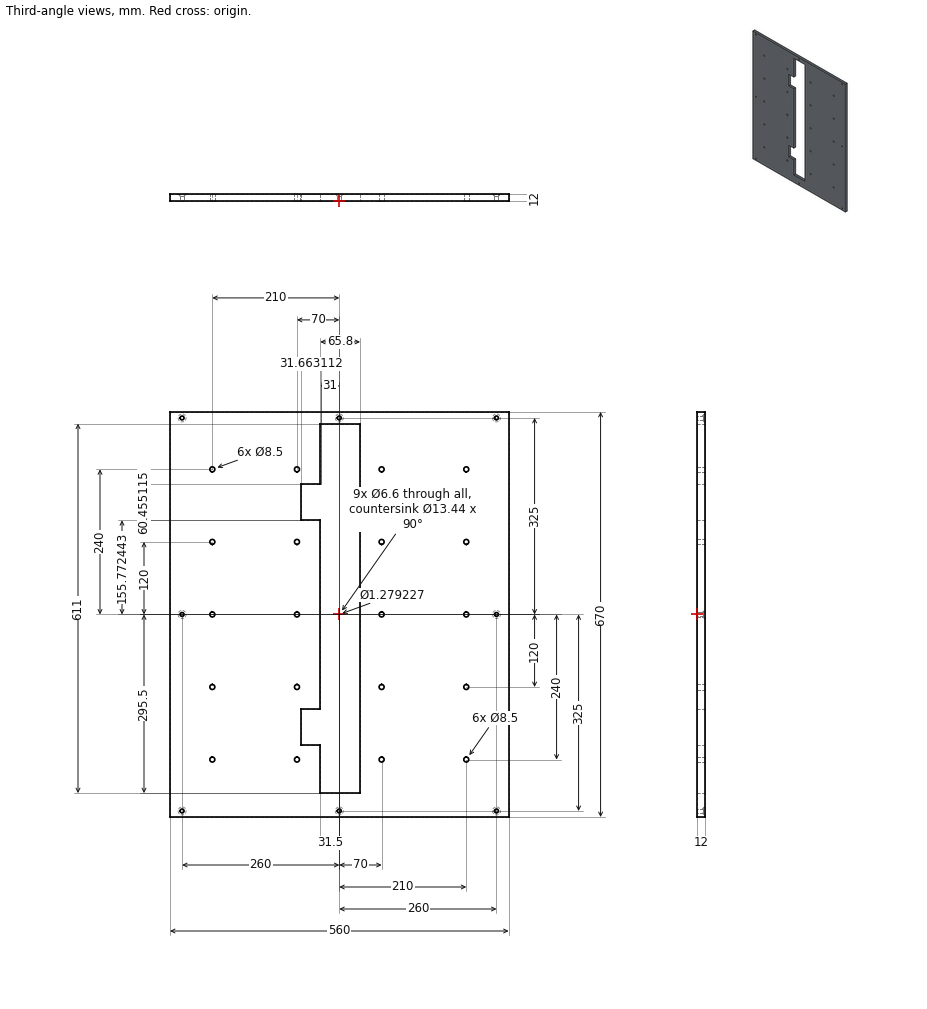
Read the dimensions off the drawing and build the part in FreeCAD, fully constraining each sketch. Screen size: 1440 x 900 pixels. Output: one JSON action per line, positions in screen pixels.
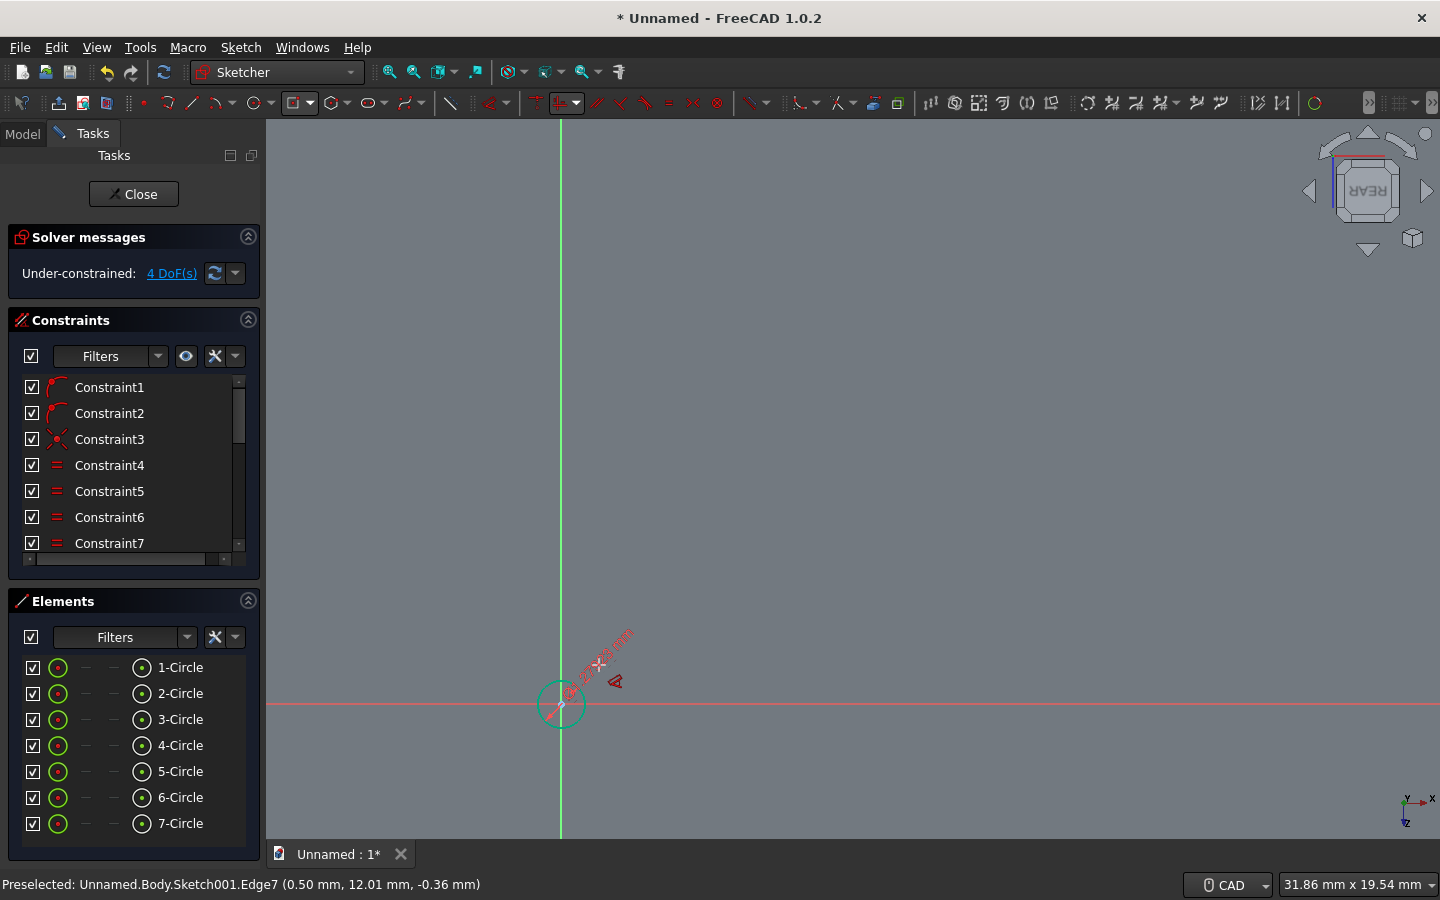
{"action": "scroll", "coordinate": [590, 699], "scroll_direction": "down", "scroll_amount": 15}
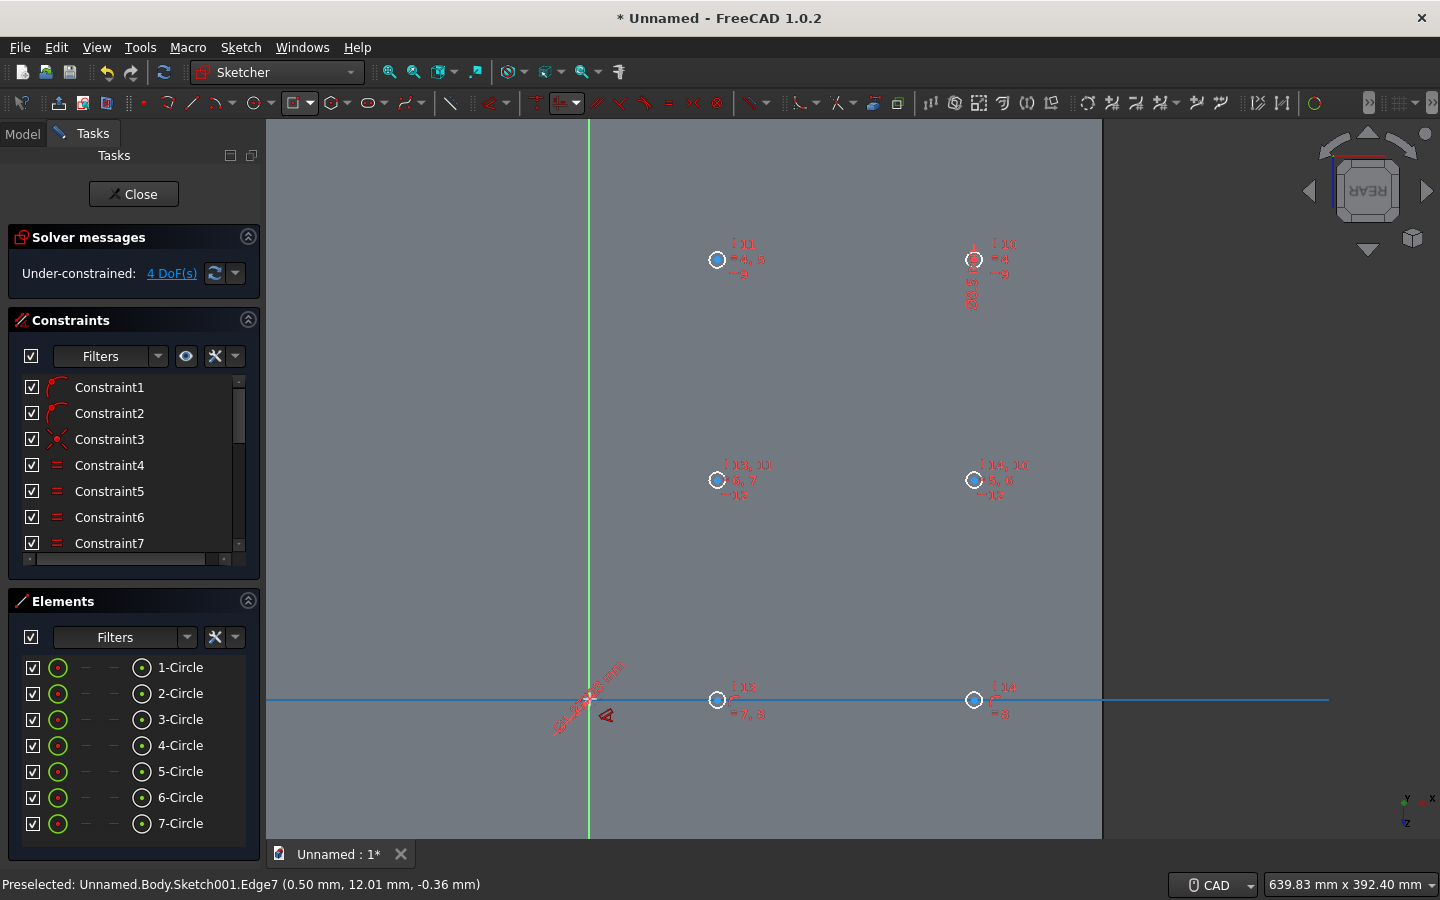
{"action": "left_click", "coordinate": [717, 260]}
{"action": "left_click", "coordinate": [653, 734]}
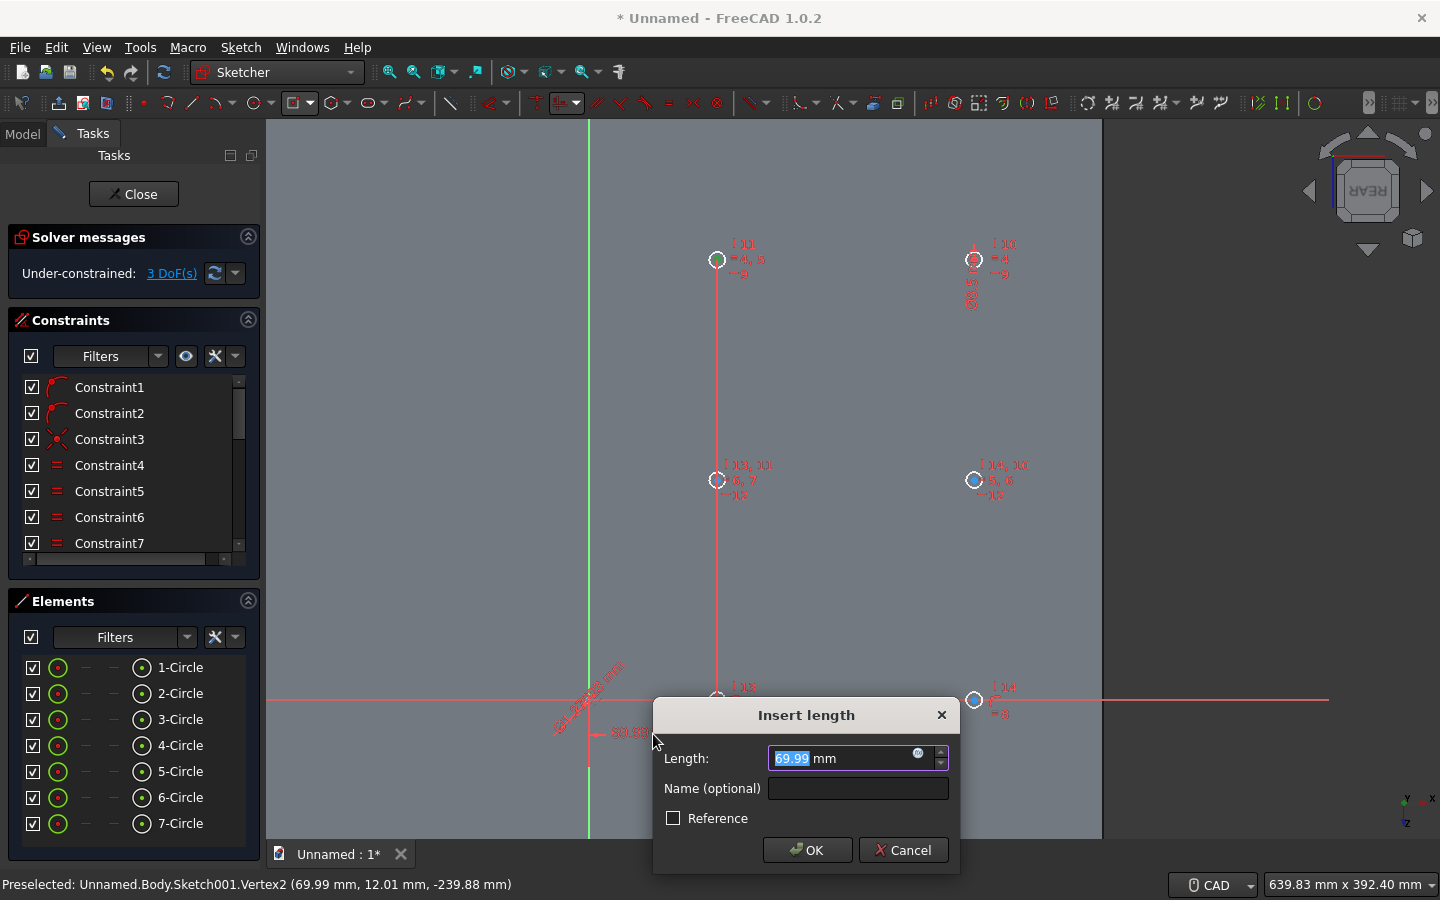
{"action": "type", "text": "70"}
{"action": "key", "text": "Return"}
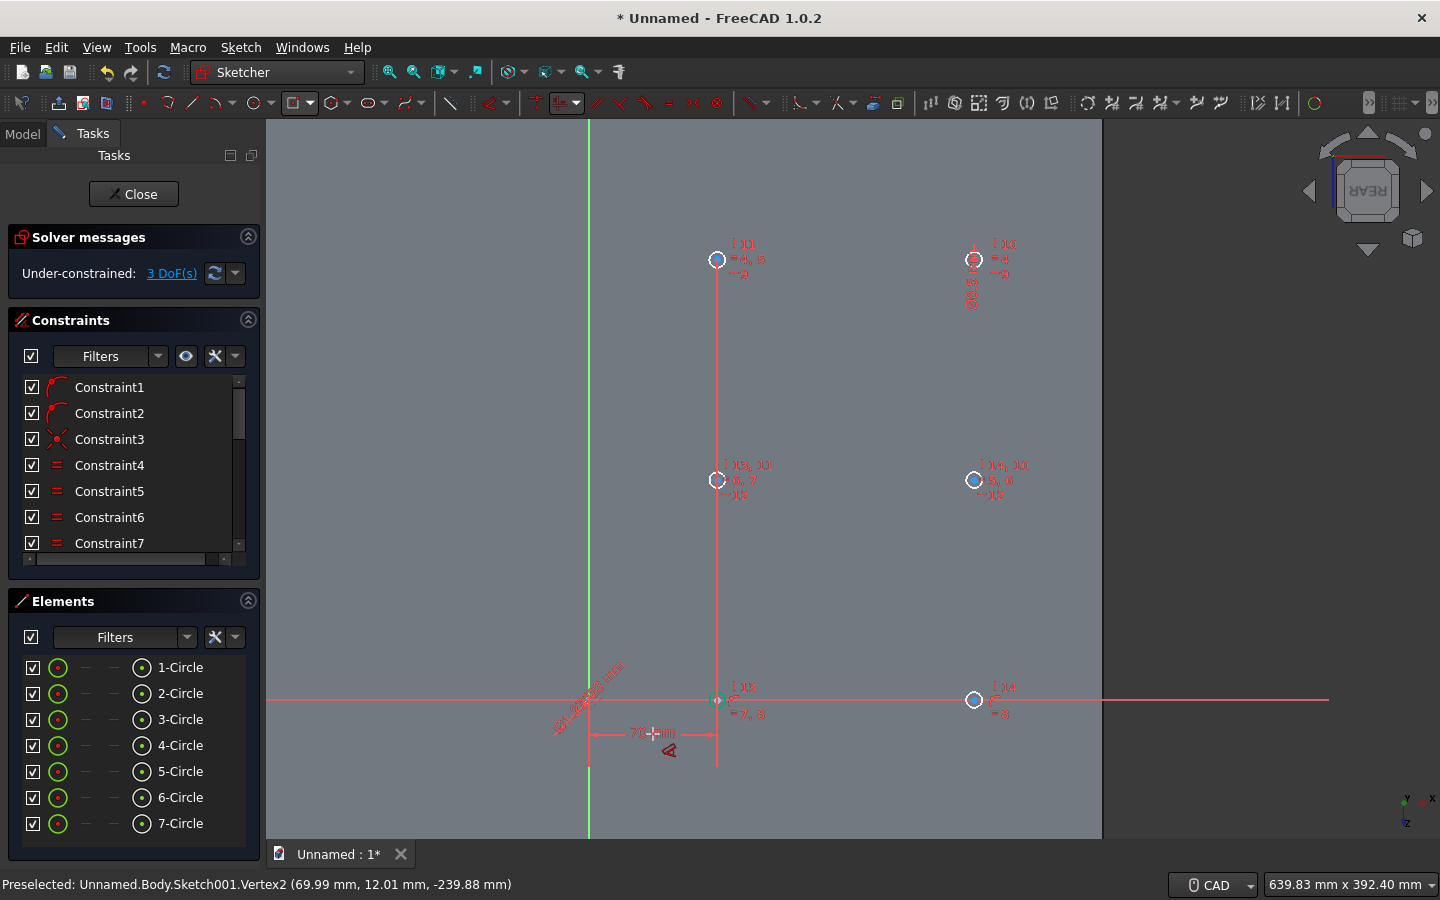
{"action": "left_click", "coordinate": [974, 260]}
{"action": "left_click", "coordinate": [781, 734]}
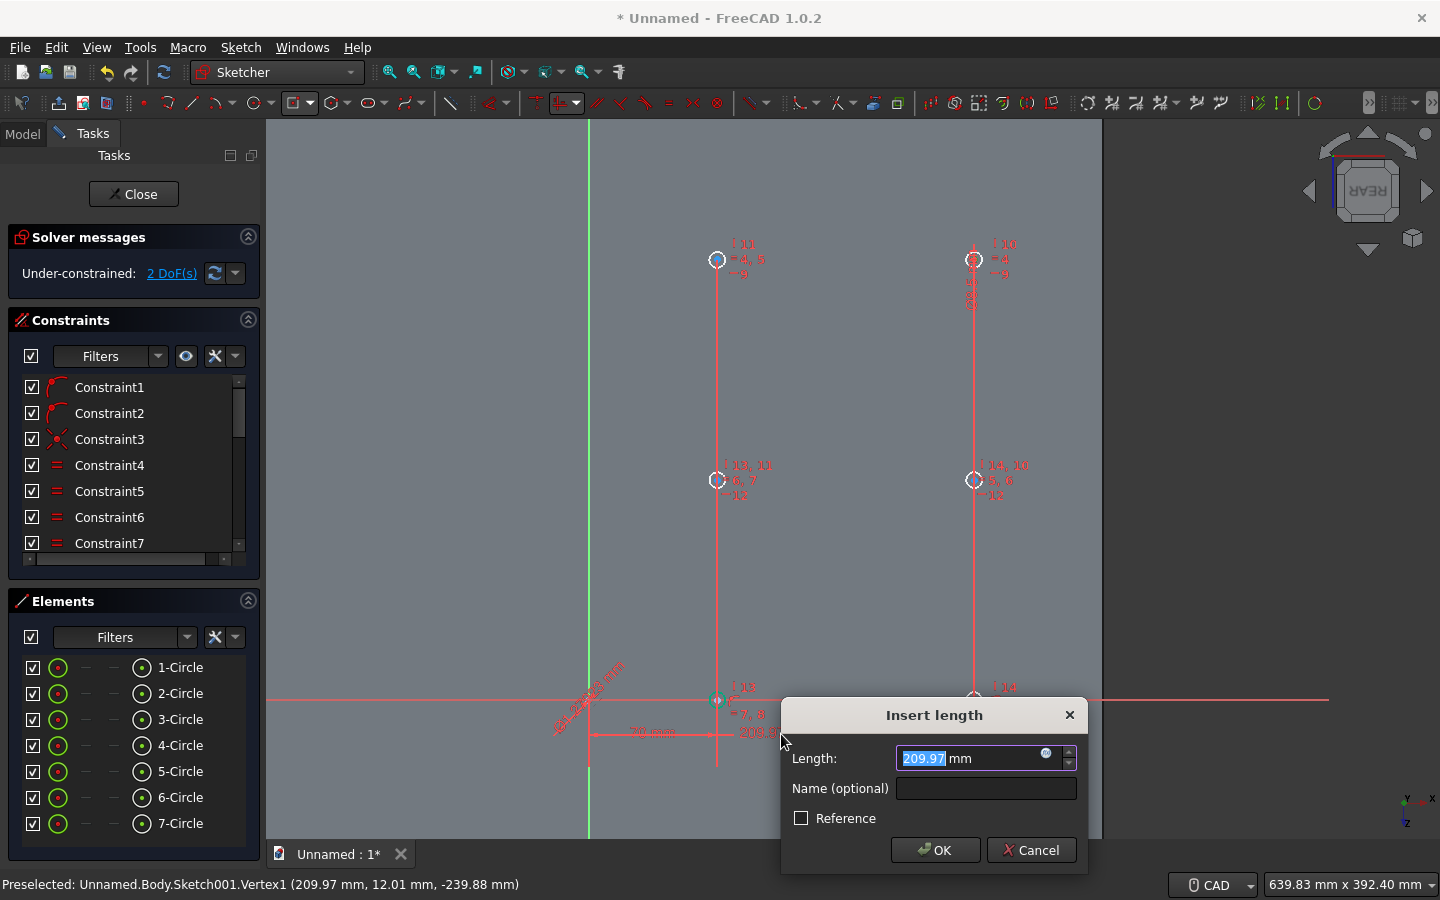
{"action": "type", "text": "210"}
{"action": "key", "text": "Return"}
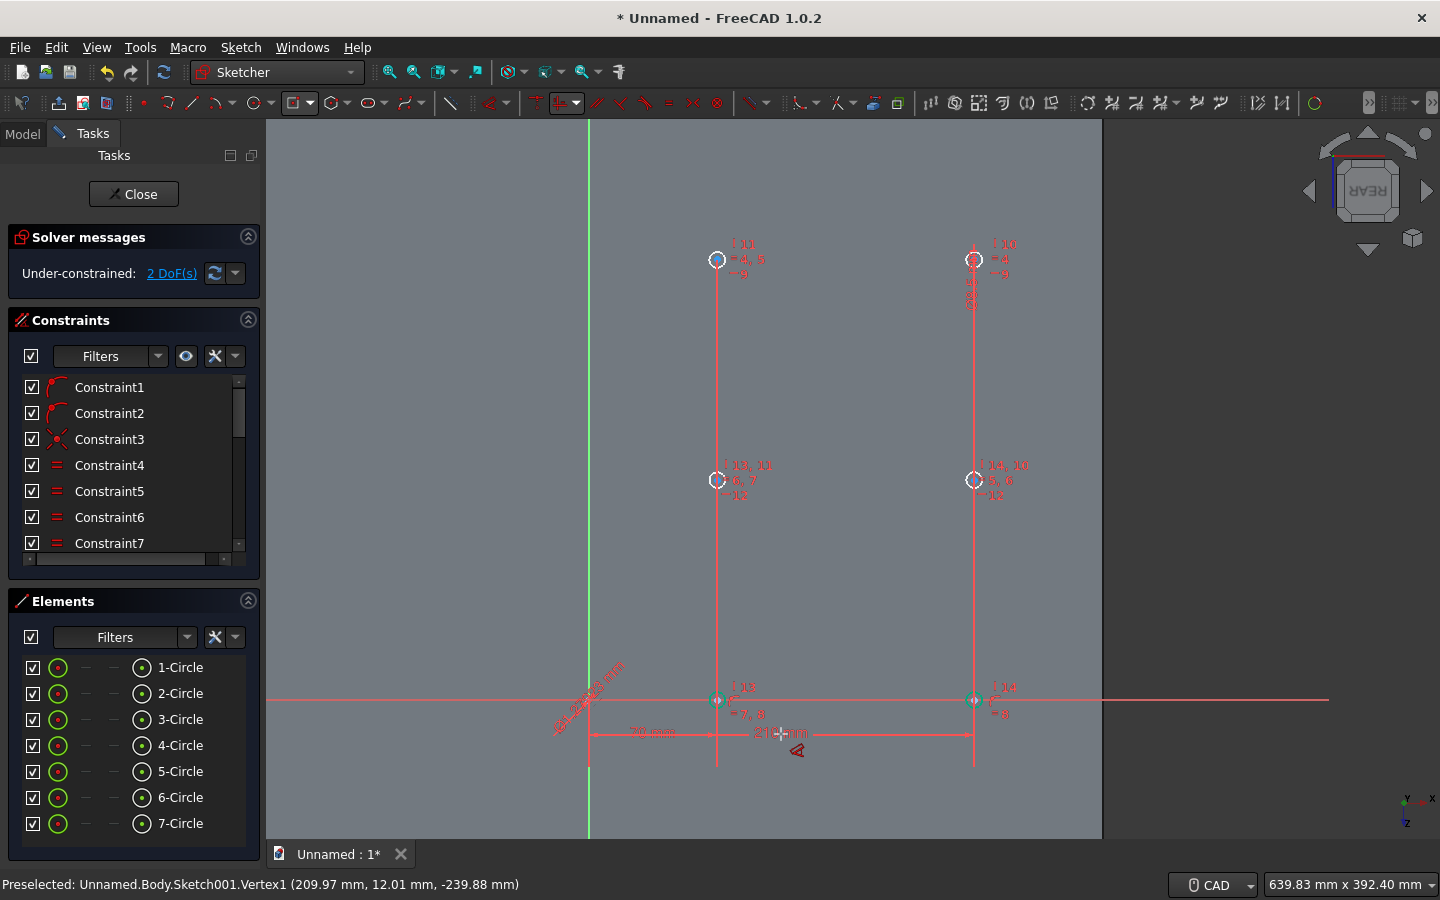
{"action": "left_click", "coordinate": [974, 260]}
{"action": "left_click", "coordinate": [555, 480]}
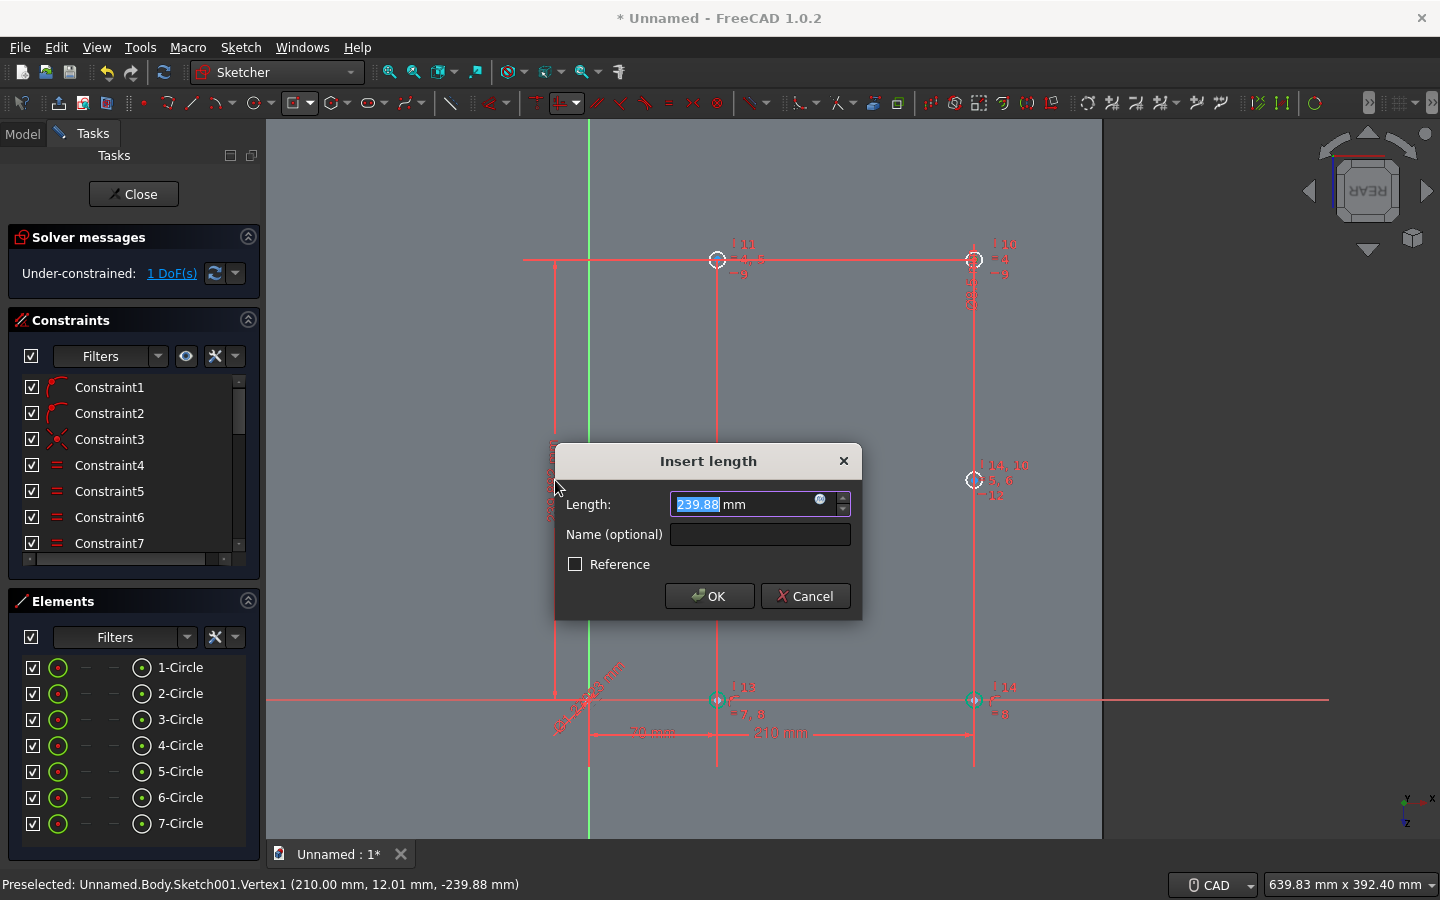
{"action": "type", "text": "240"}
{"action": "key", "text": "Return"}